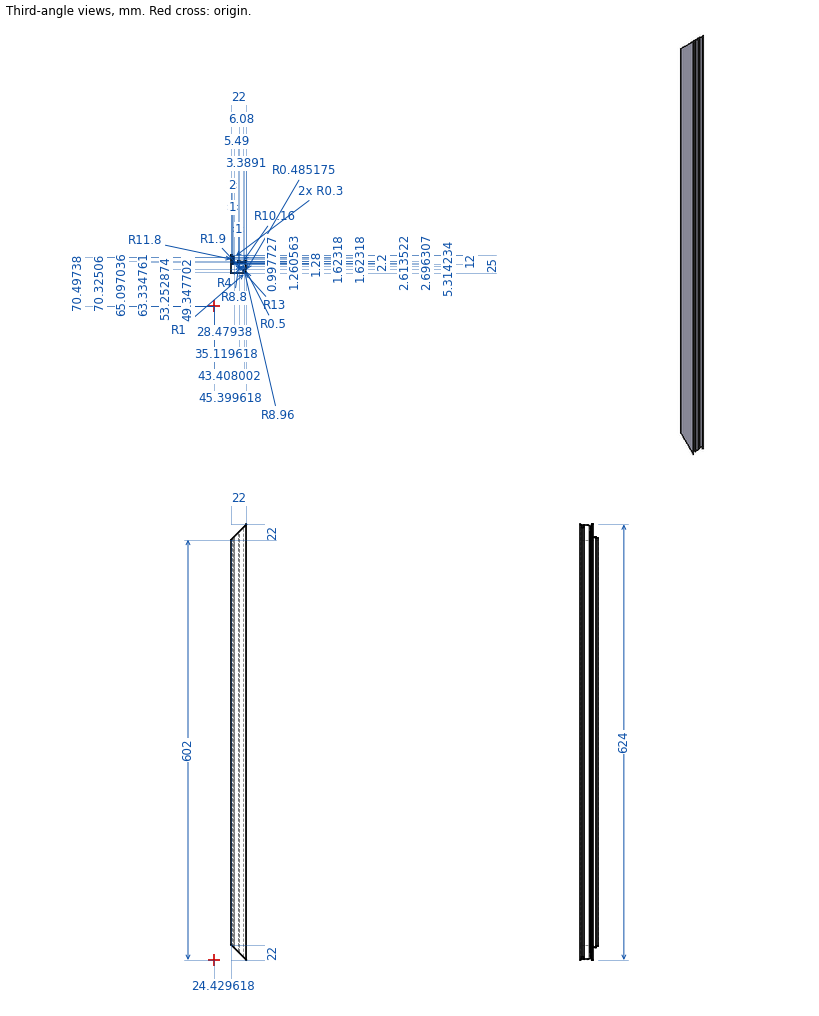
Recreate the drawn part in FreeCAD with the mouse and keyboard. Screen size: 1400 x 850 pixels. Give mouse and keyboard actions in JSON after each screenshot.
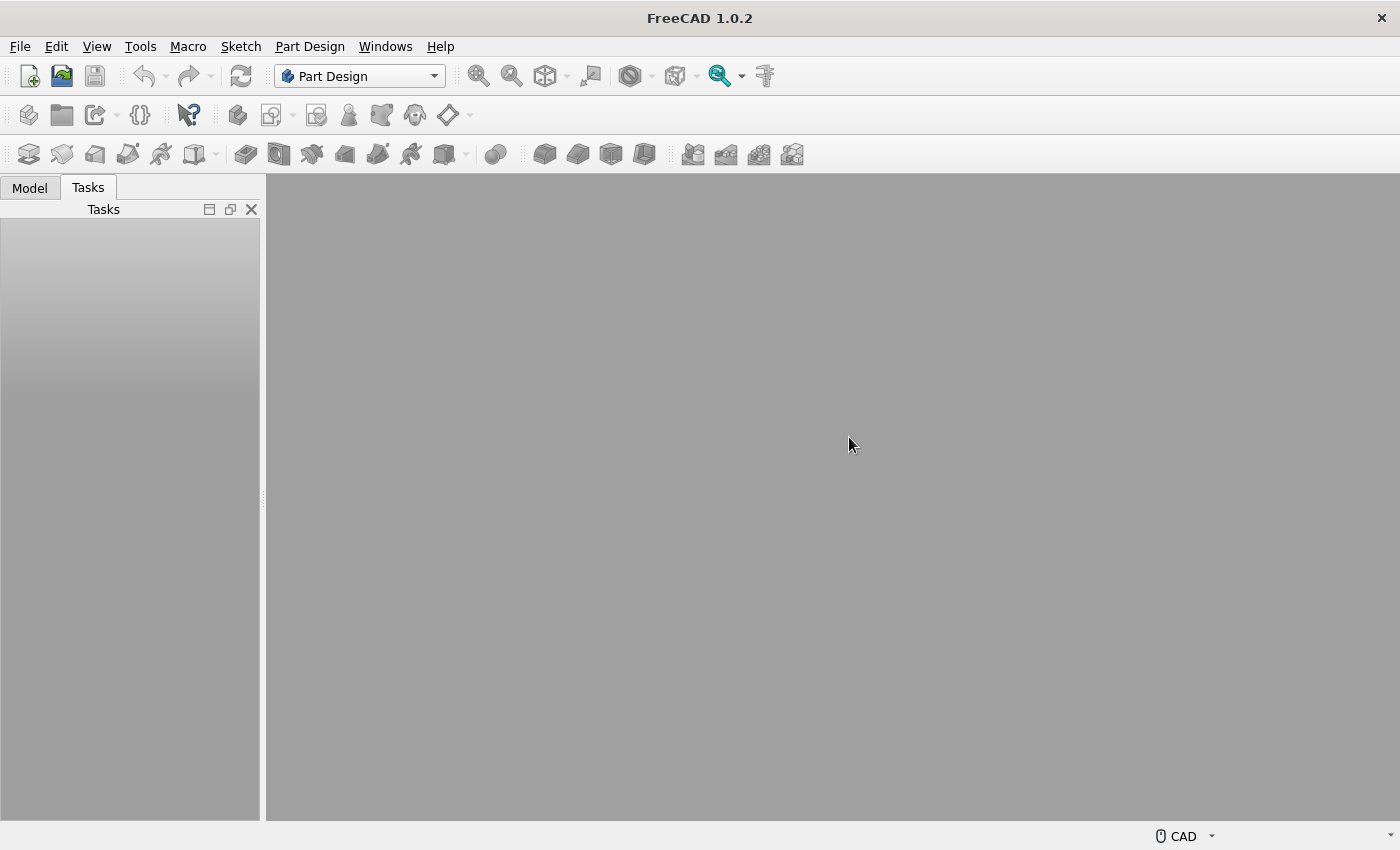
{"action": "key", "text": "ctrl+n"}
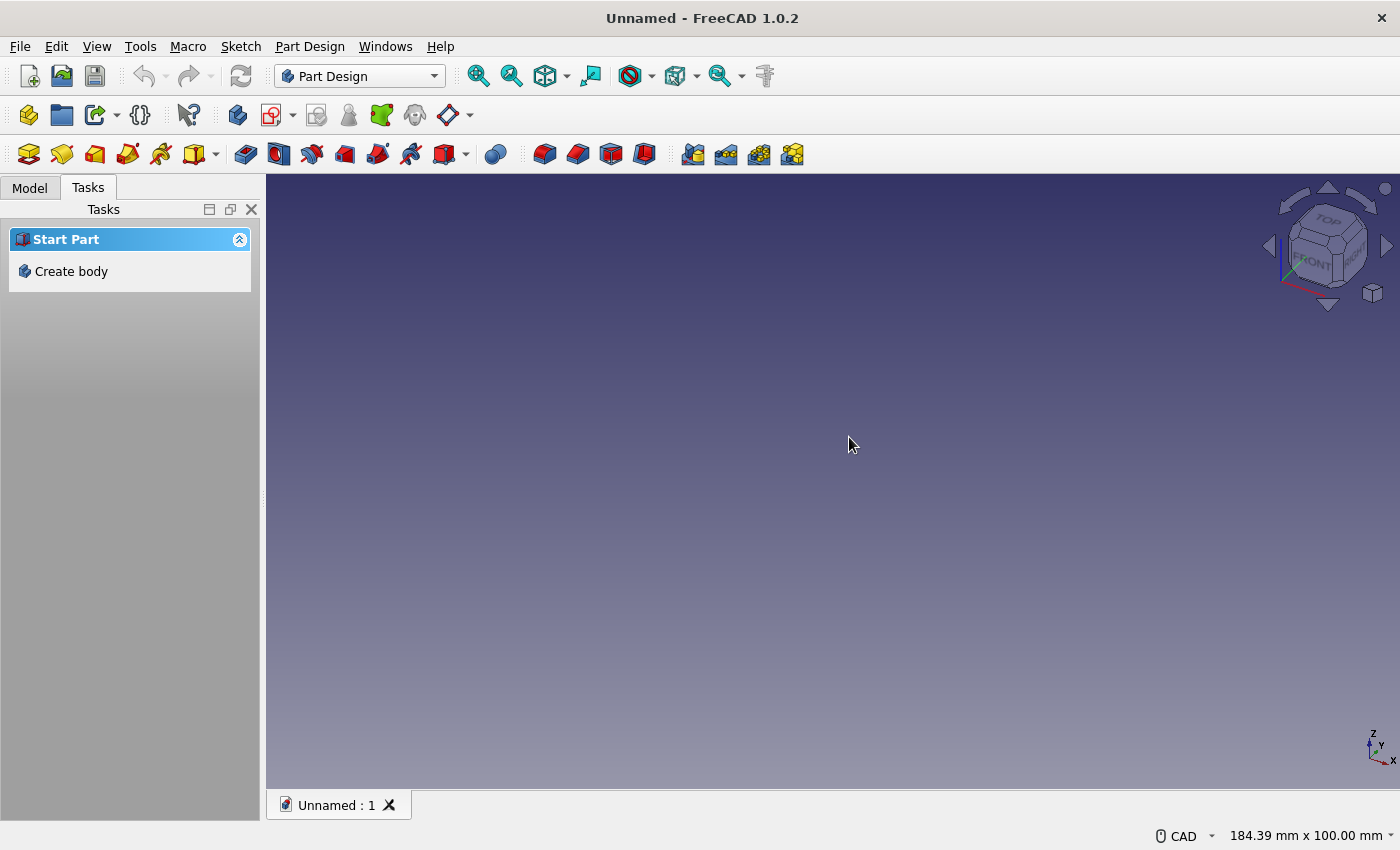
{"action": "left_click", "coordinate": [270, 116]}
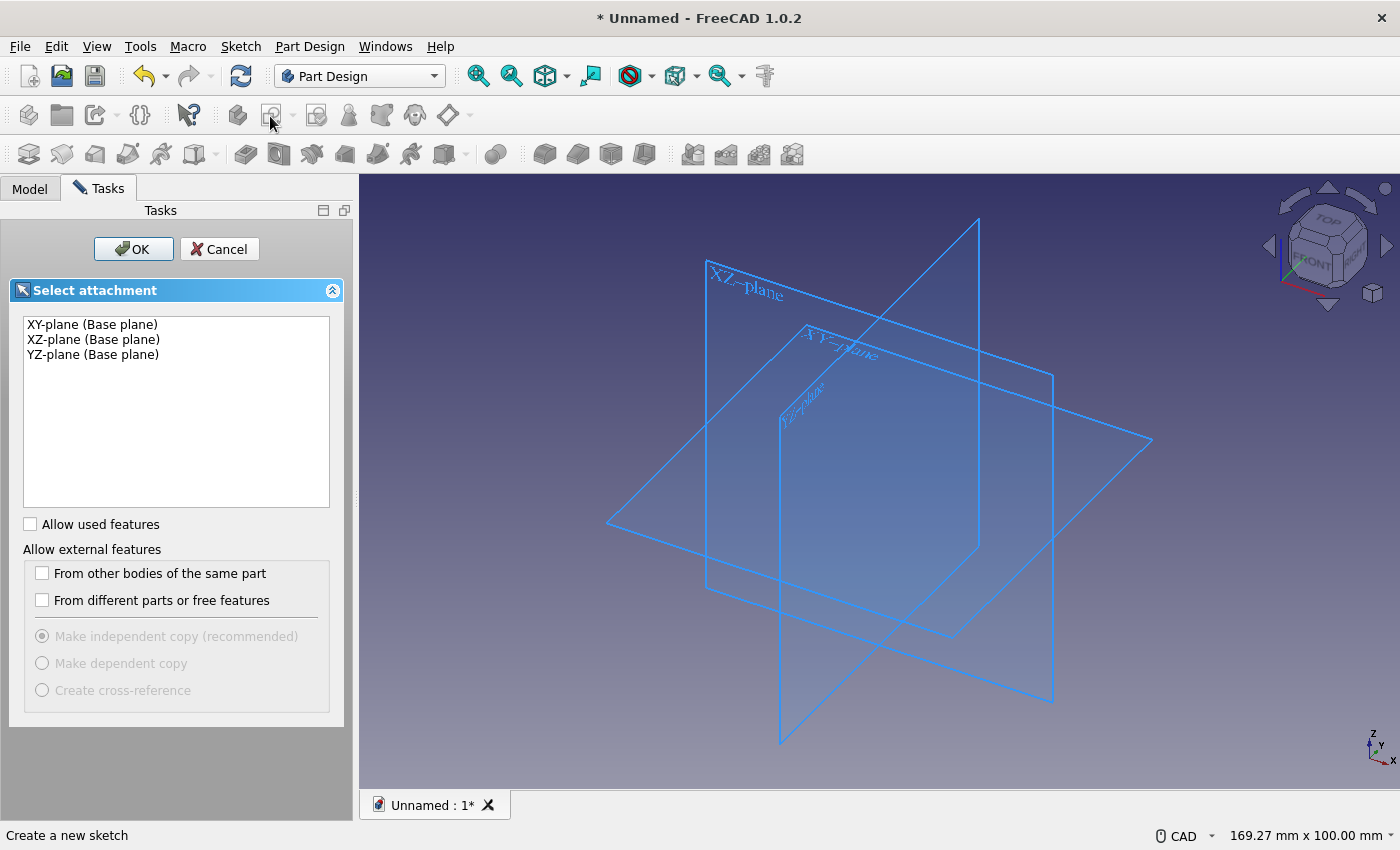
{"action": "left_click", "coordinate": [84, 324]}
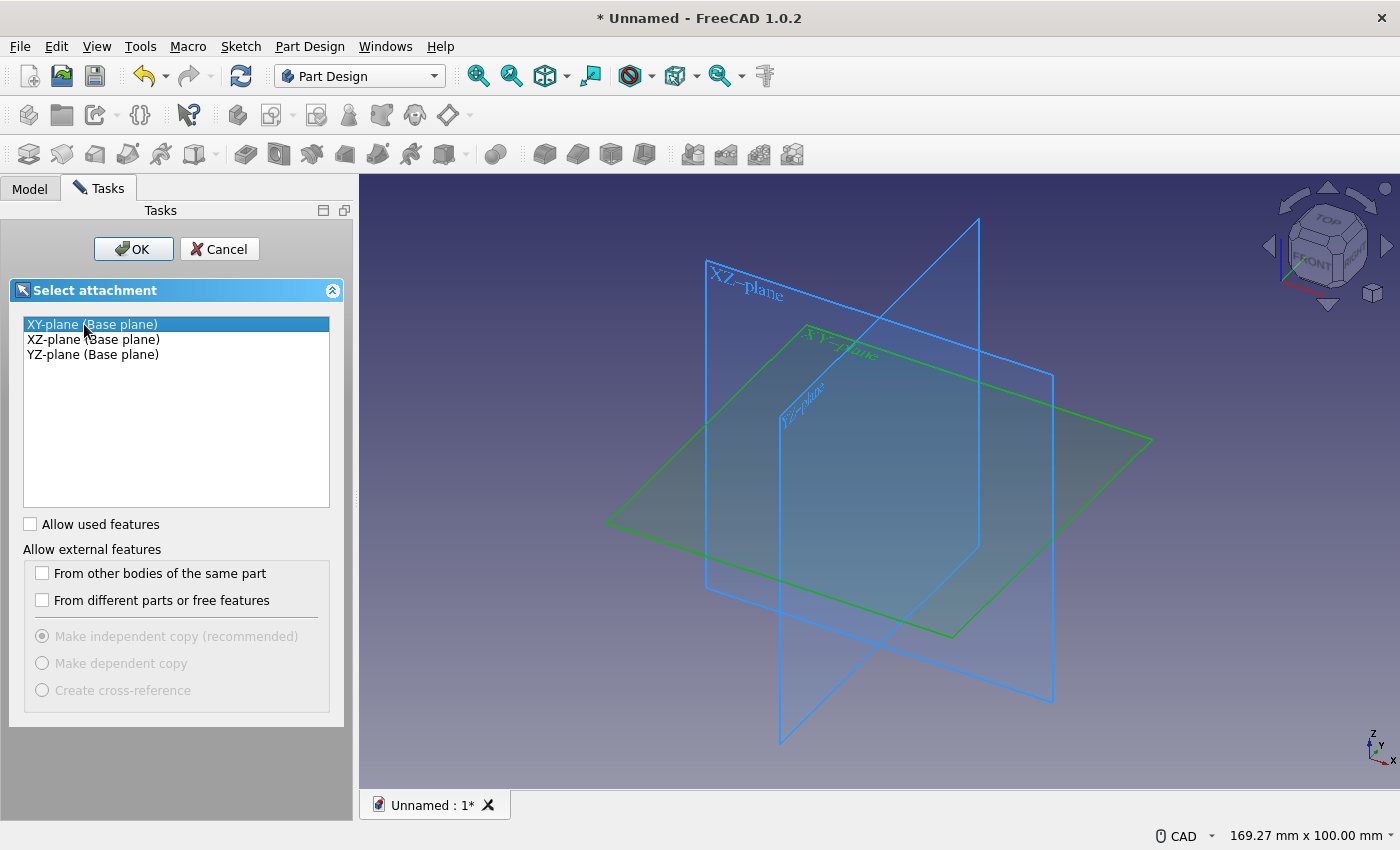
{"action": "left_click", "coordinate": [134, 249]}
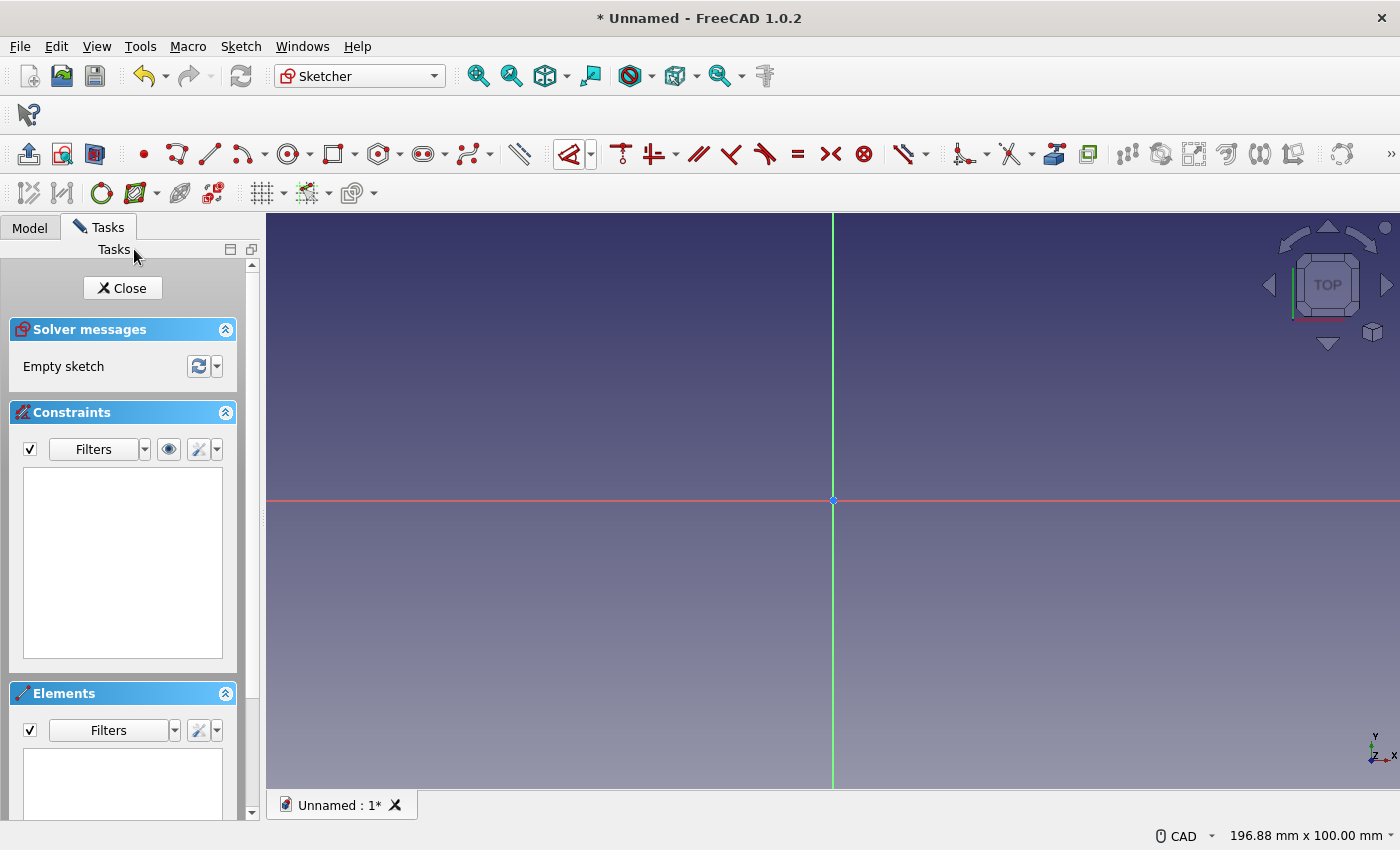
{"action": "scroll", "coordinate": [764, 501], "scroll_direction": "down", "scroll_amount": 5}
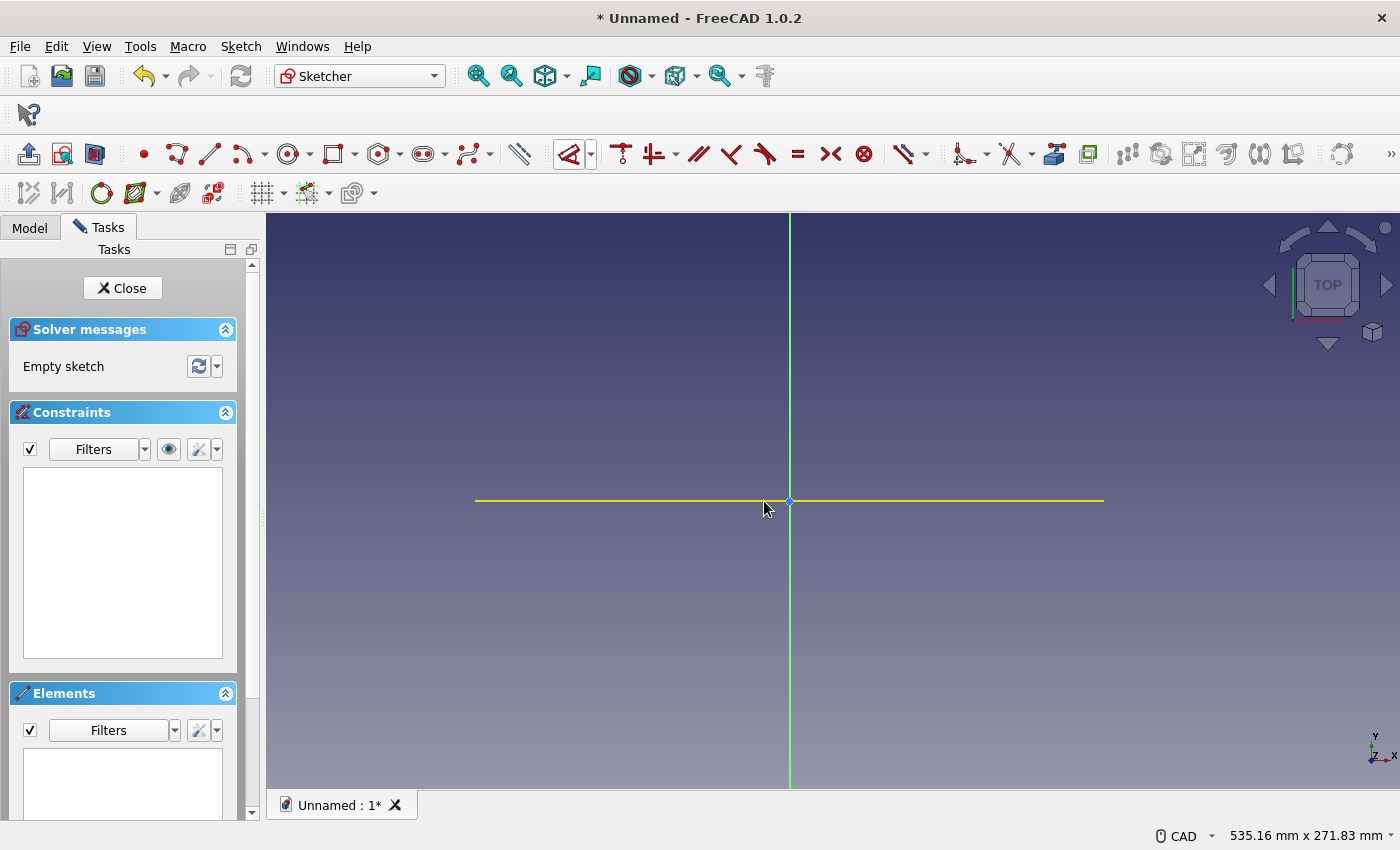
{"action": "scroll", "coordinate": [880, 353], "scroll_direction": "up", "scroll_amount": 10}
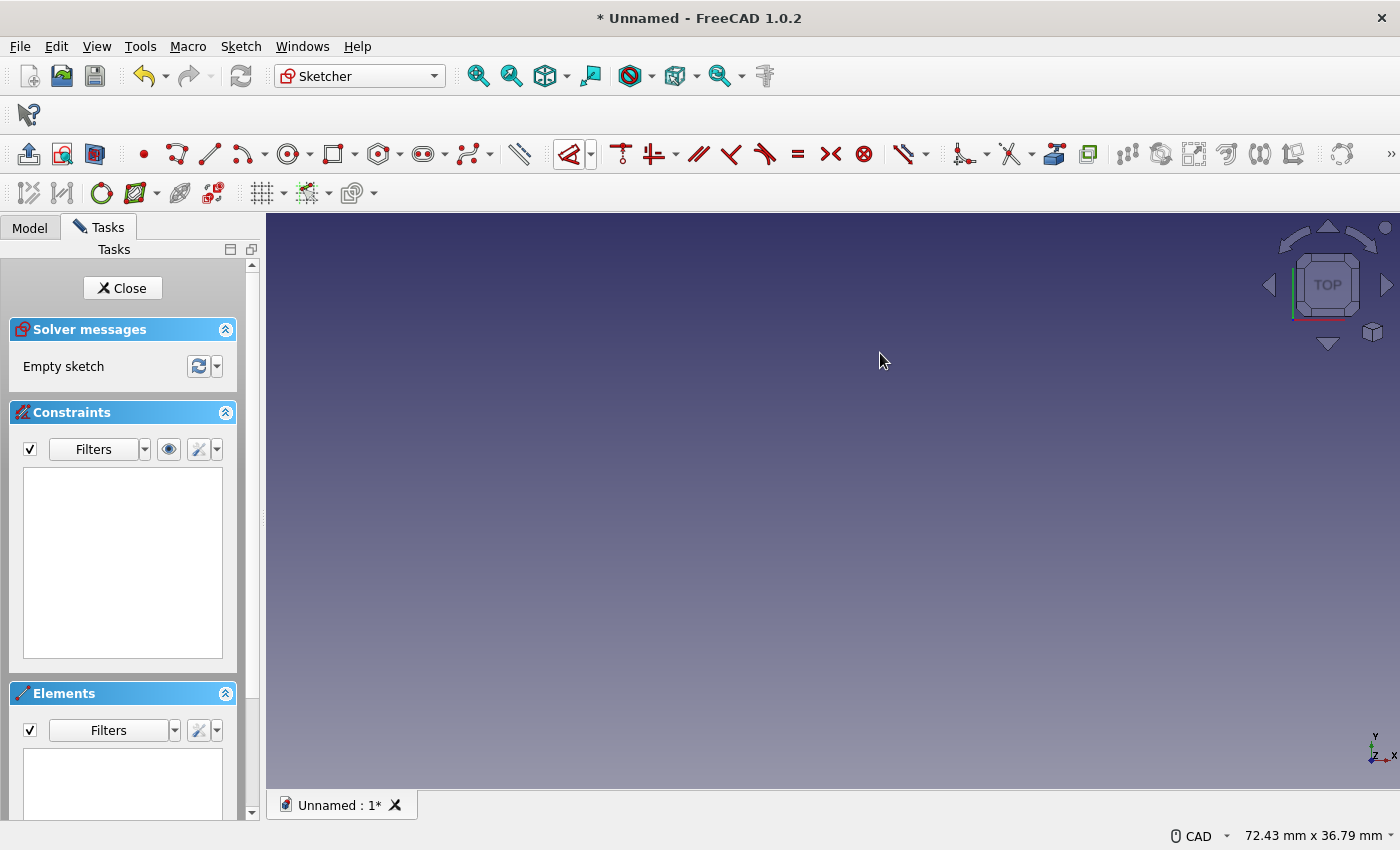
{"action": "key", "text": "g l"}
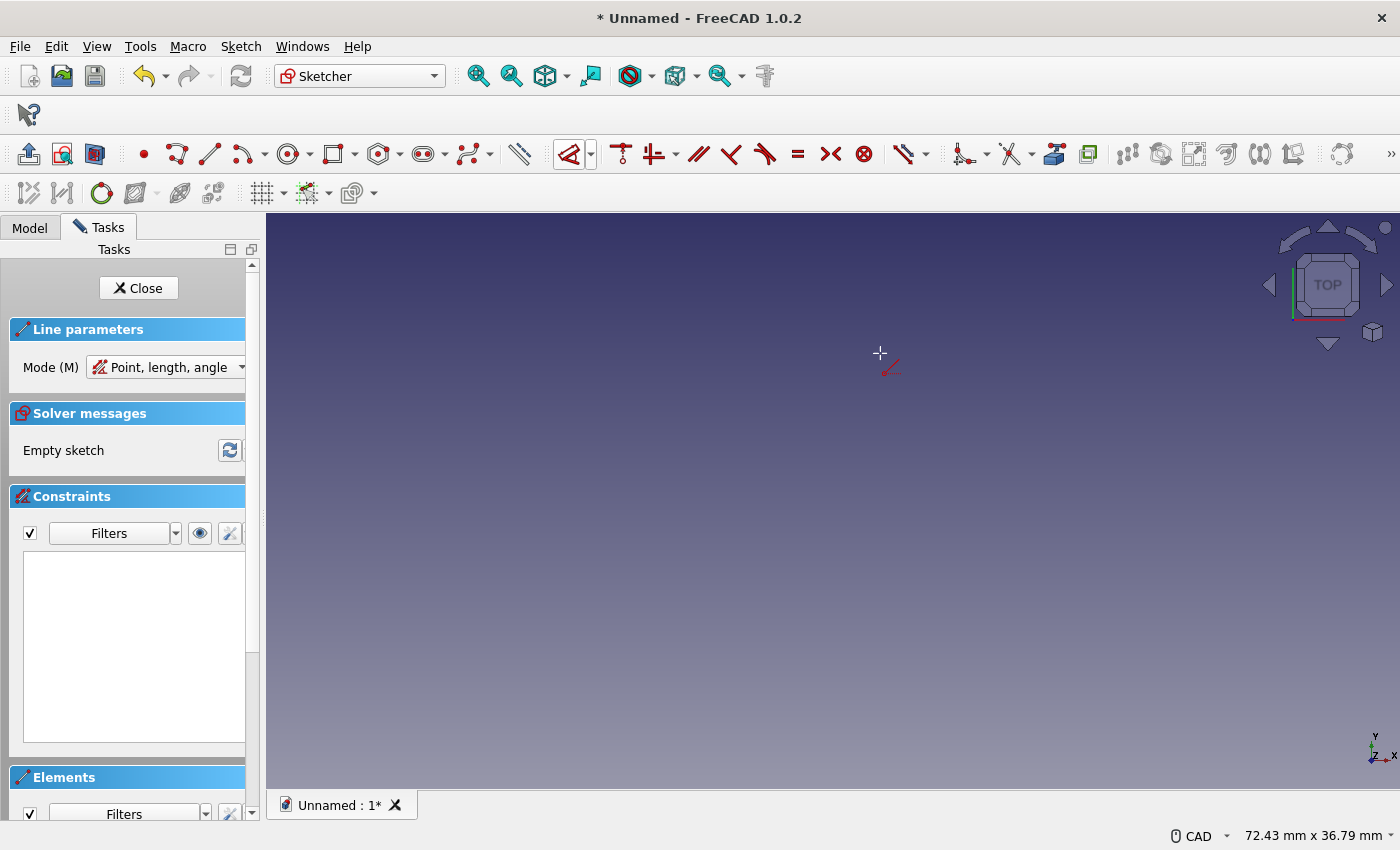
{"action": "left_click", "coordinate": [920, 614]}
{"action": "left_click", "coordinate": [920, 530]}